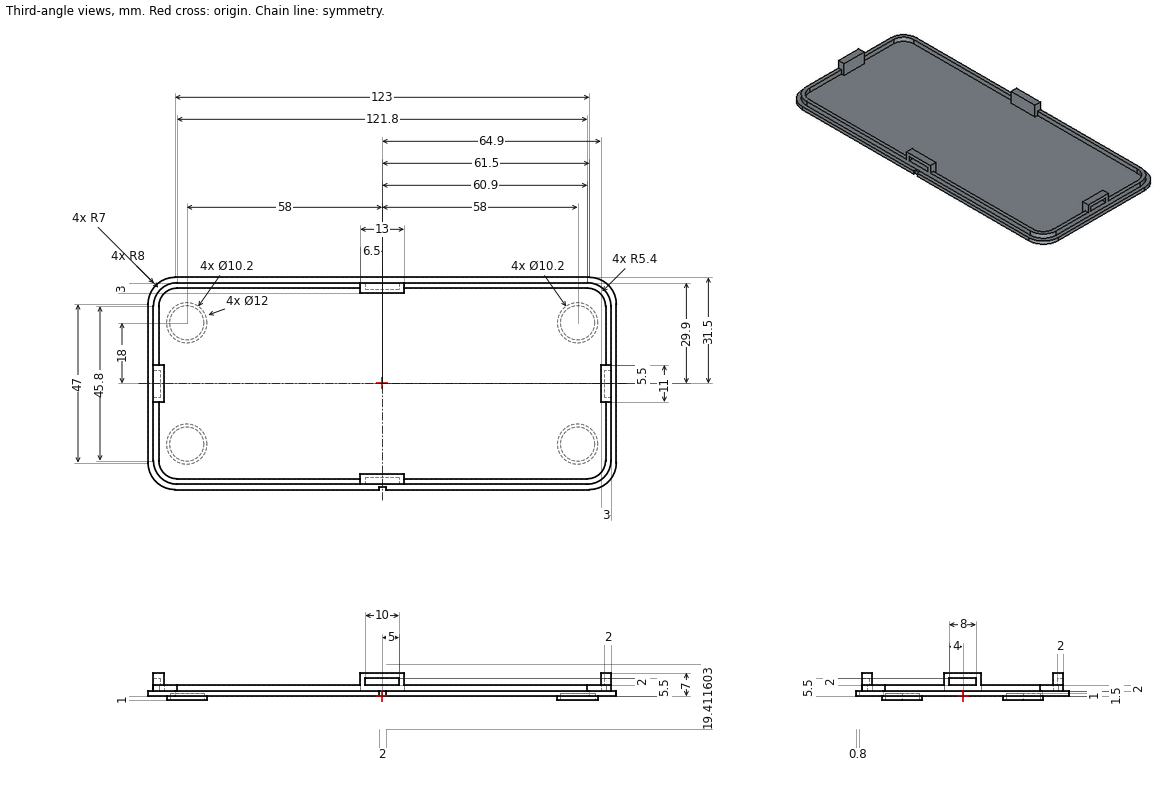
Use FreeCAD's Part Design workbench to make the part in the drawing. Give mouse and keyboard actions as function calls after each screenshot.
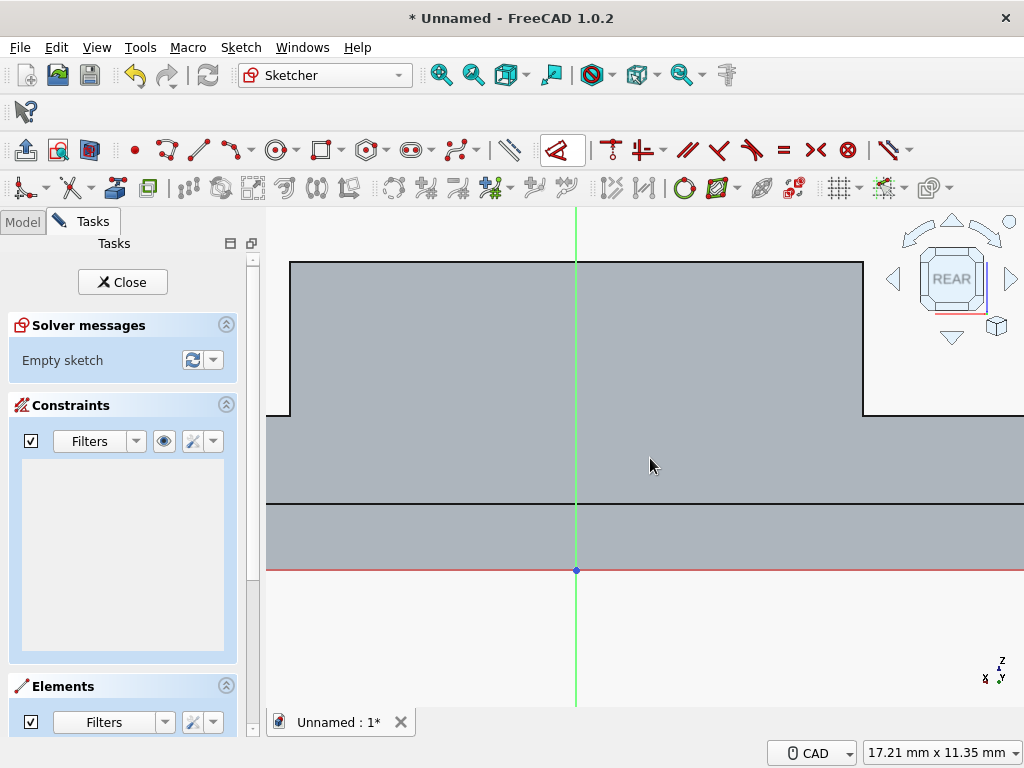
key(g)
key(r)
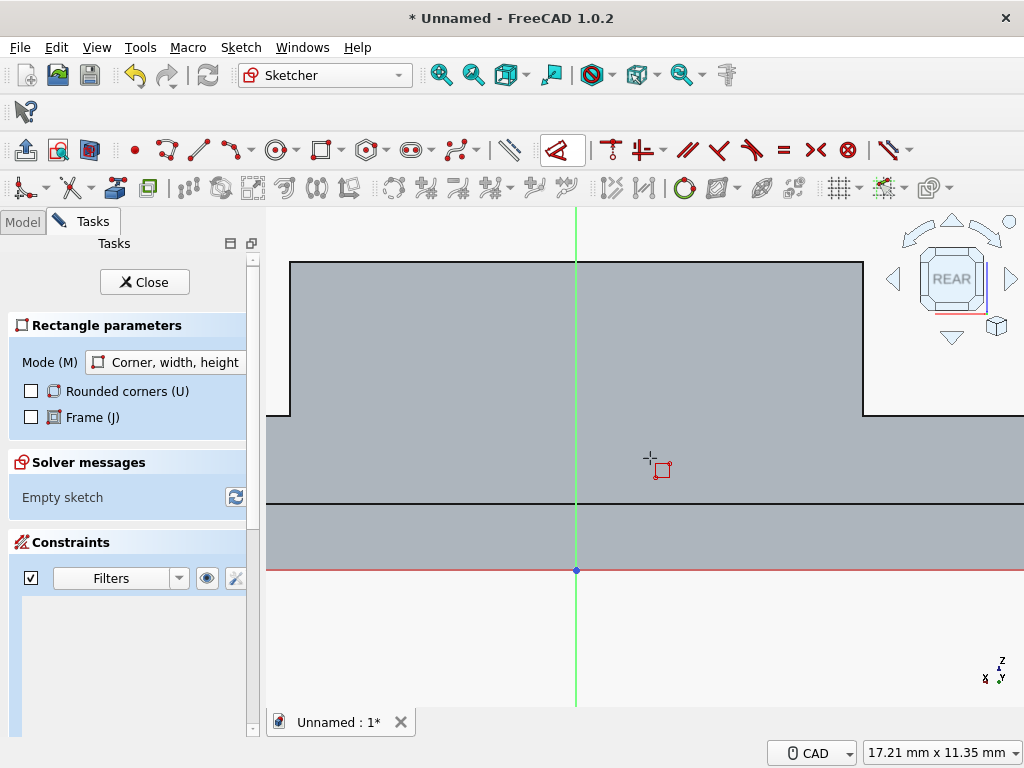
click(356, 328)
click(797, 416)
key(Escape)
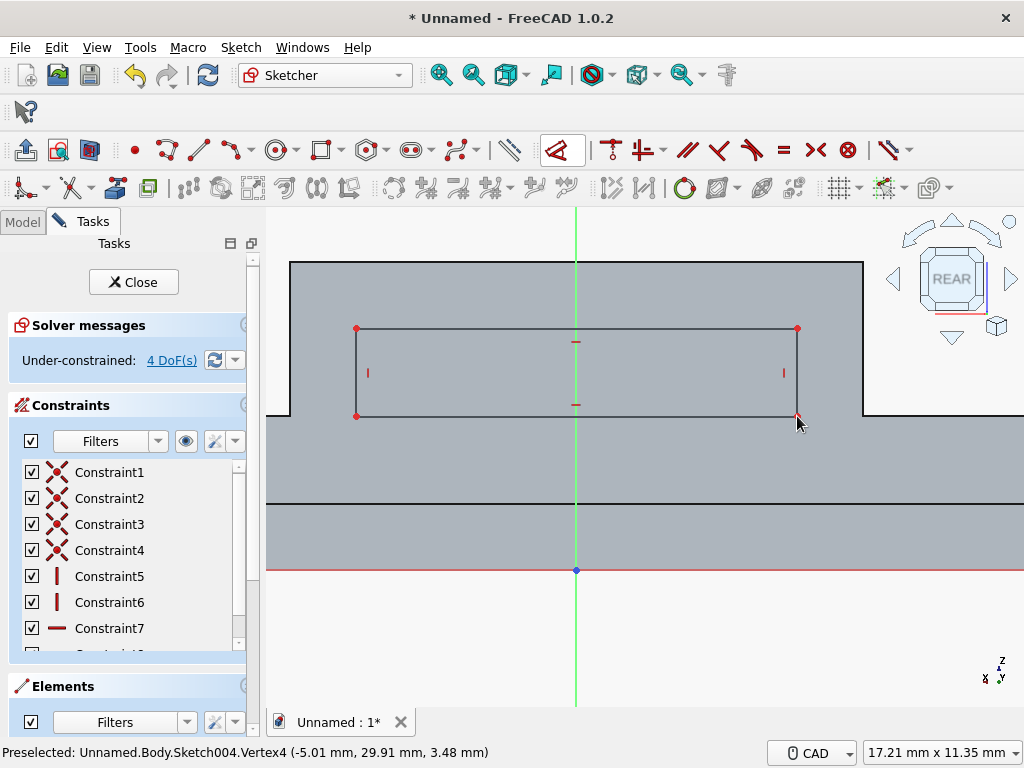
click(356, 355)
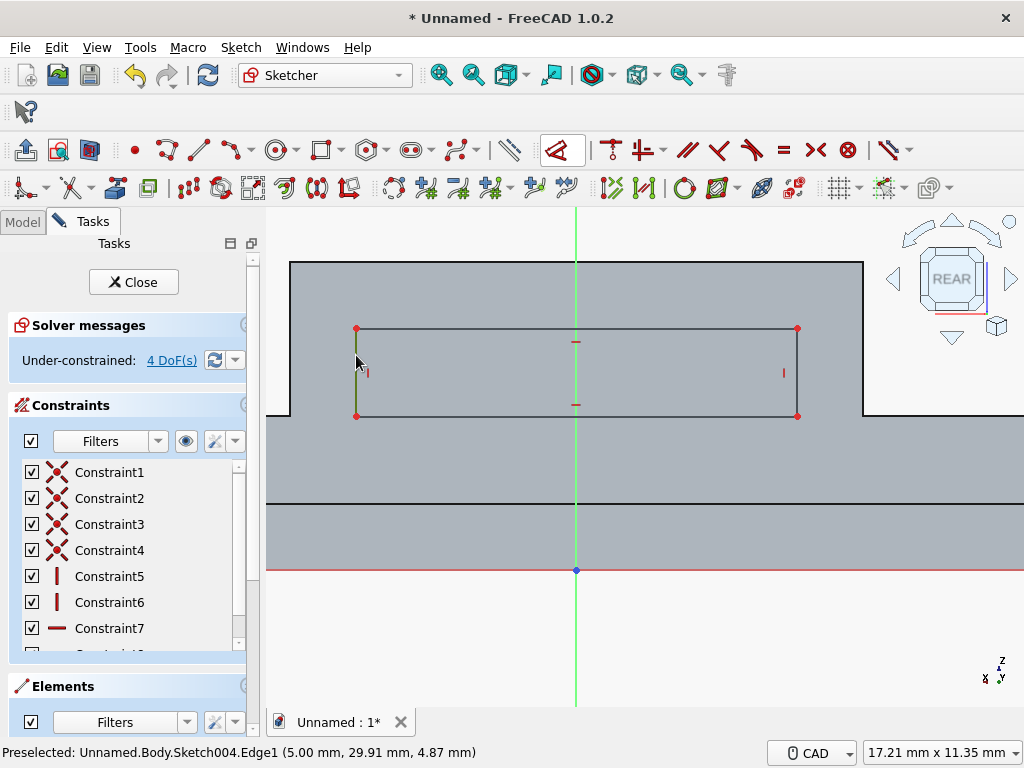
key(i)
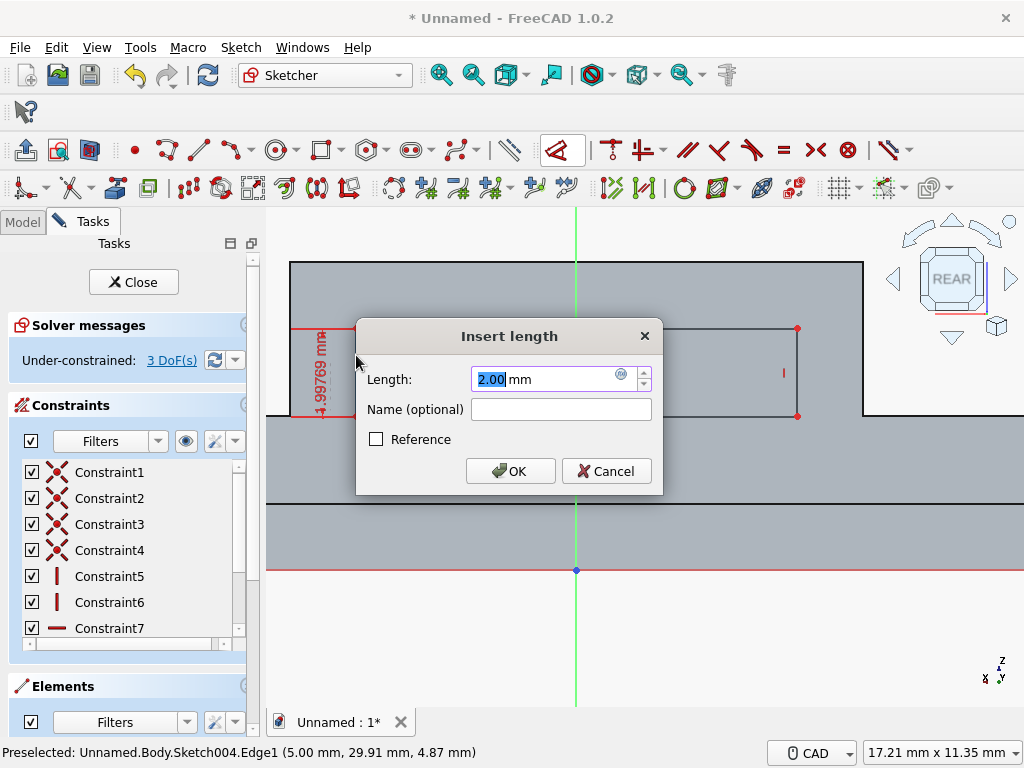
text(2)
key(Return)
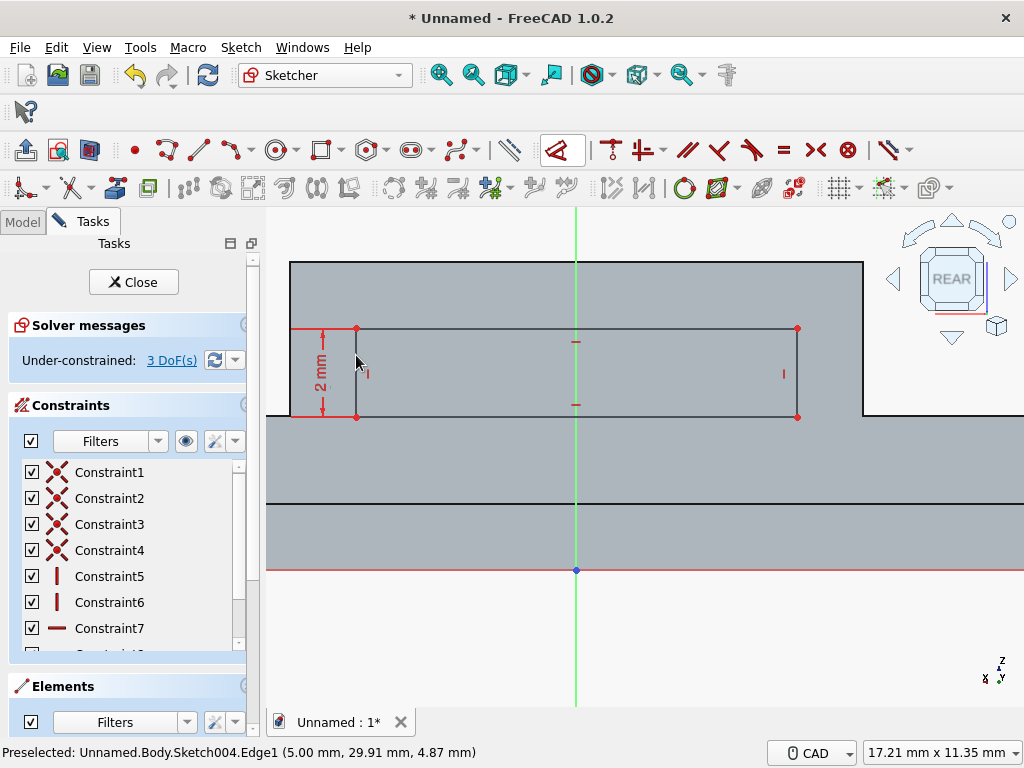
click(488, 417)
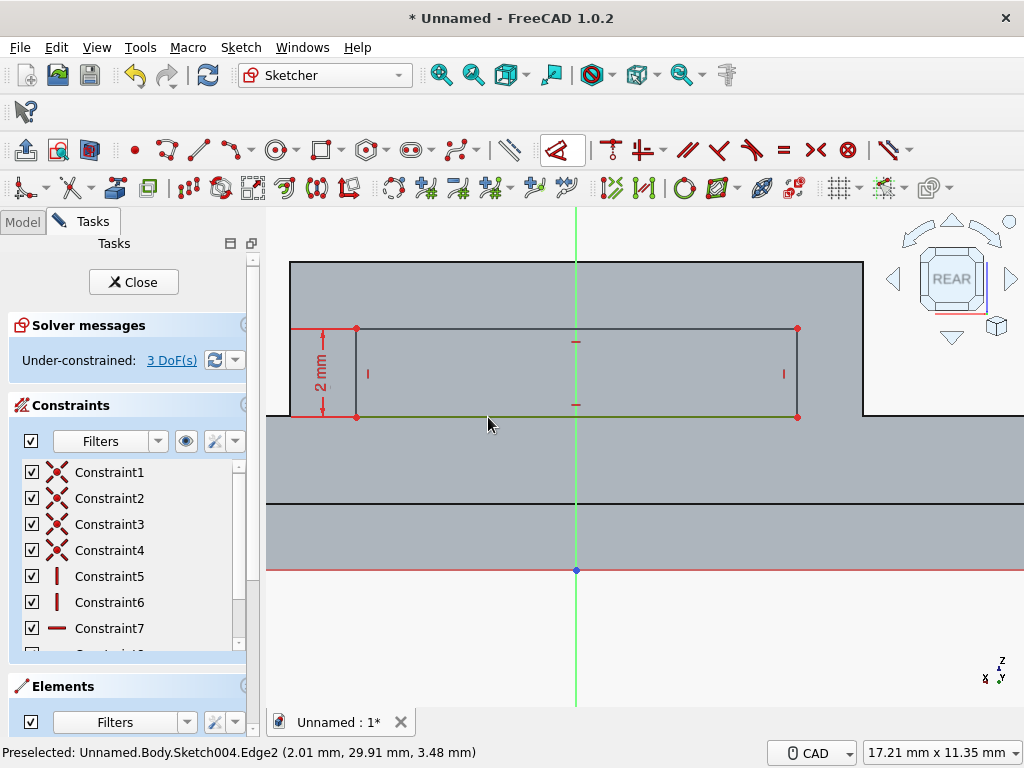
key(l)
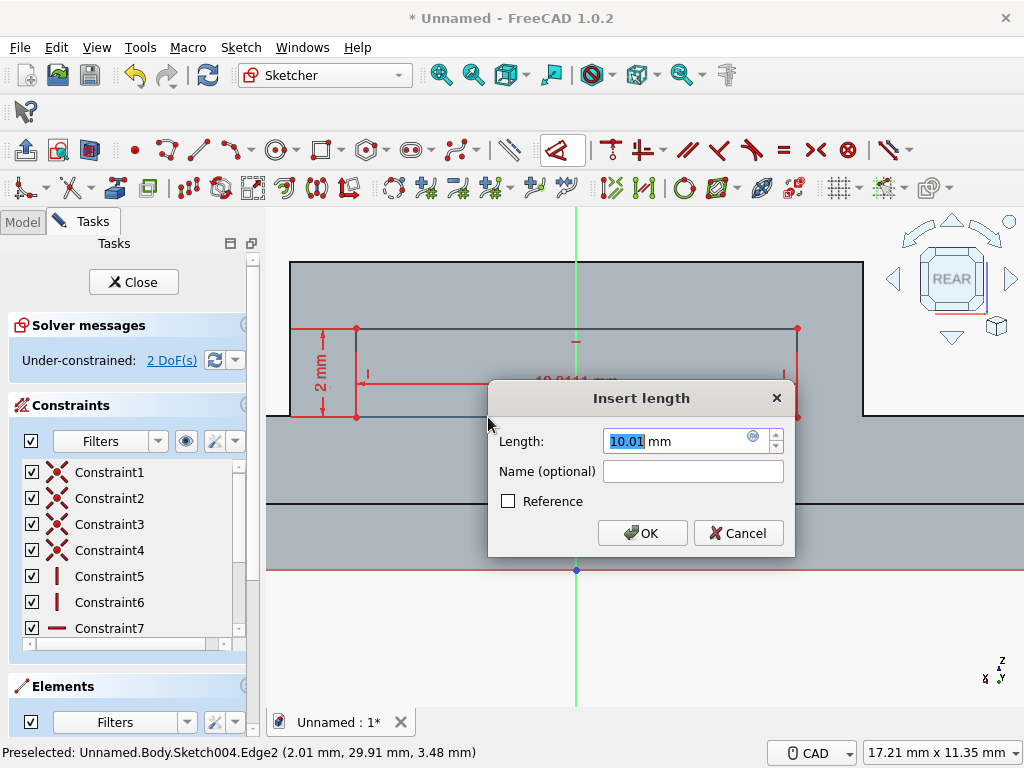
text(10)
key(Return)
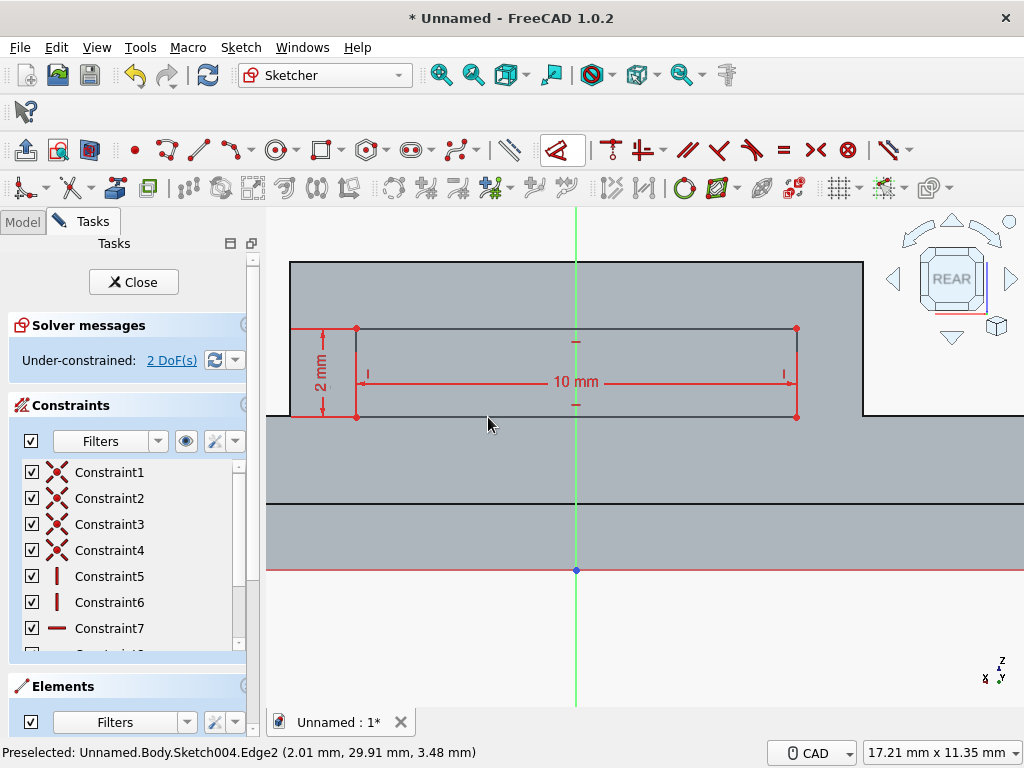
click(356, 329)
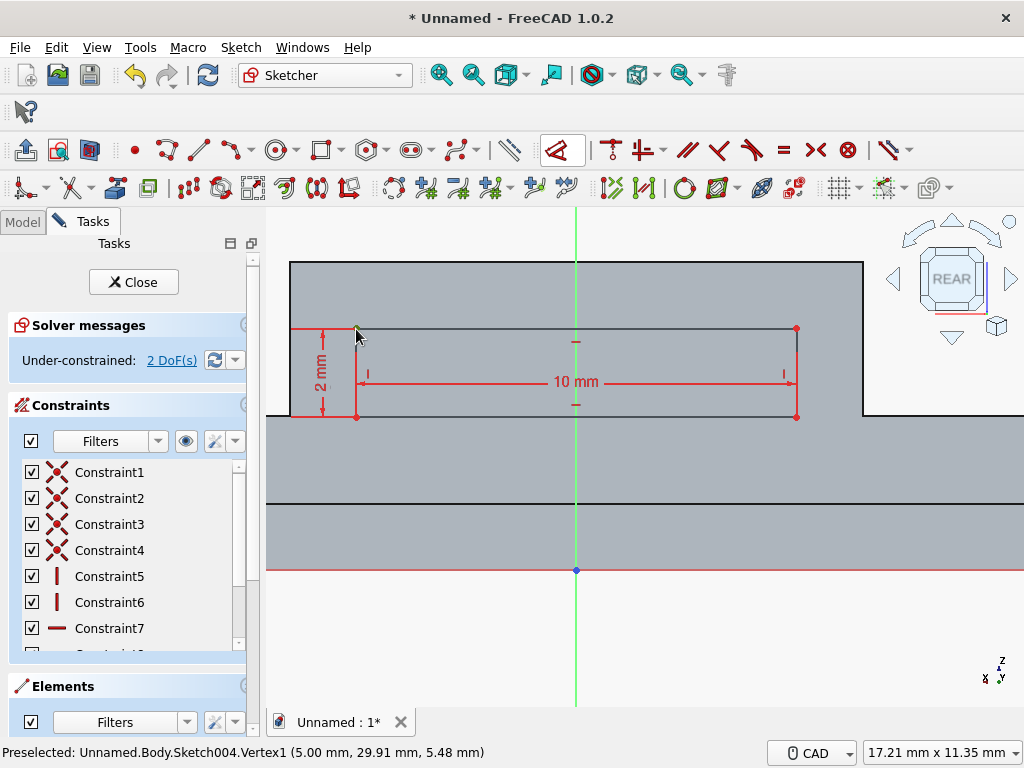
key(l)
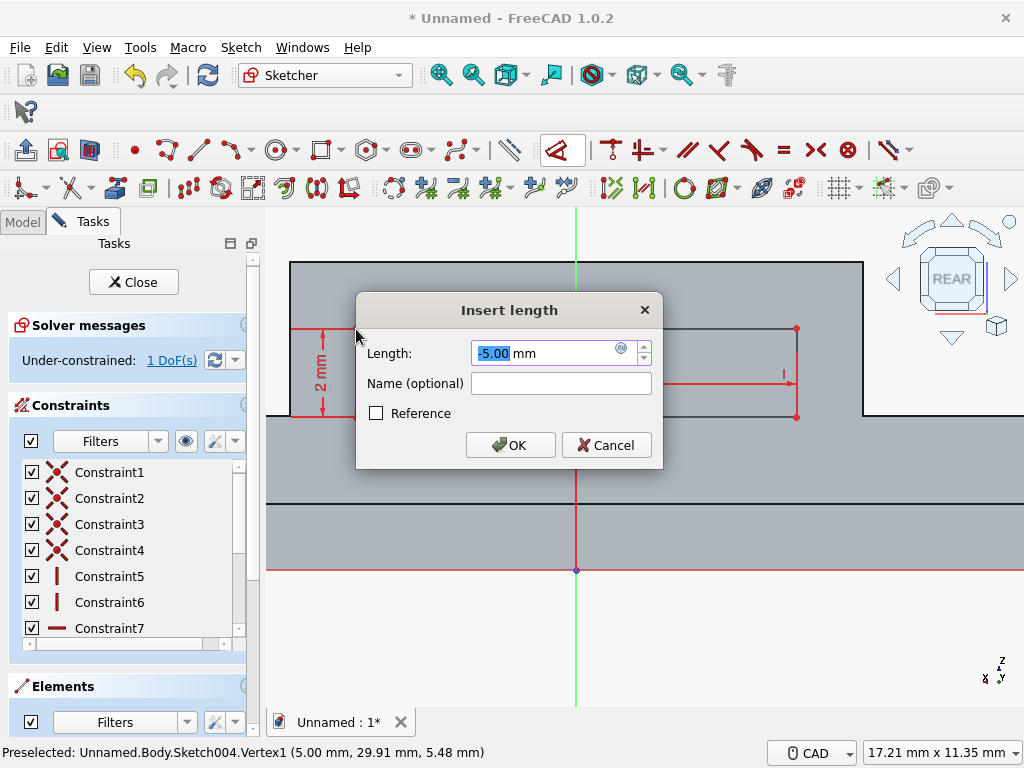
text(-5)
key(Return)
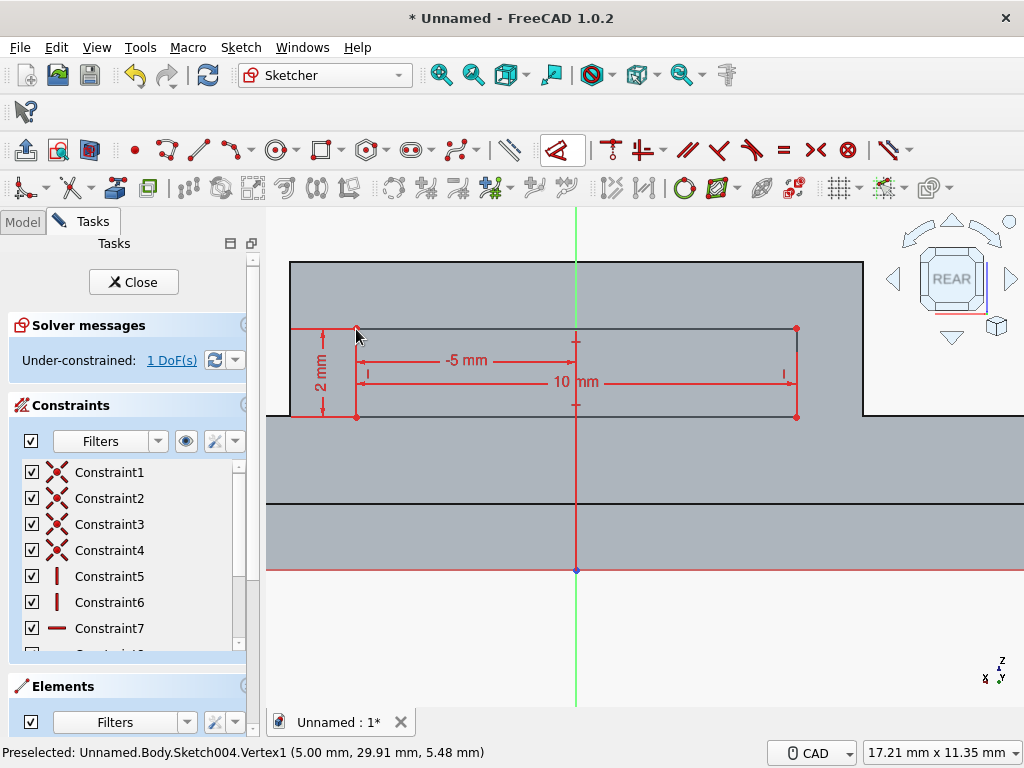
click(356, 329)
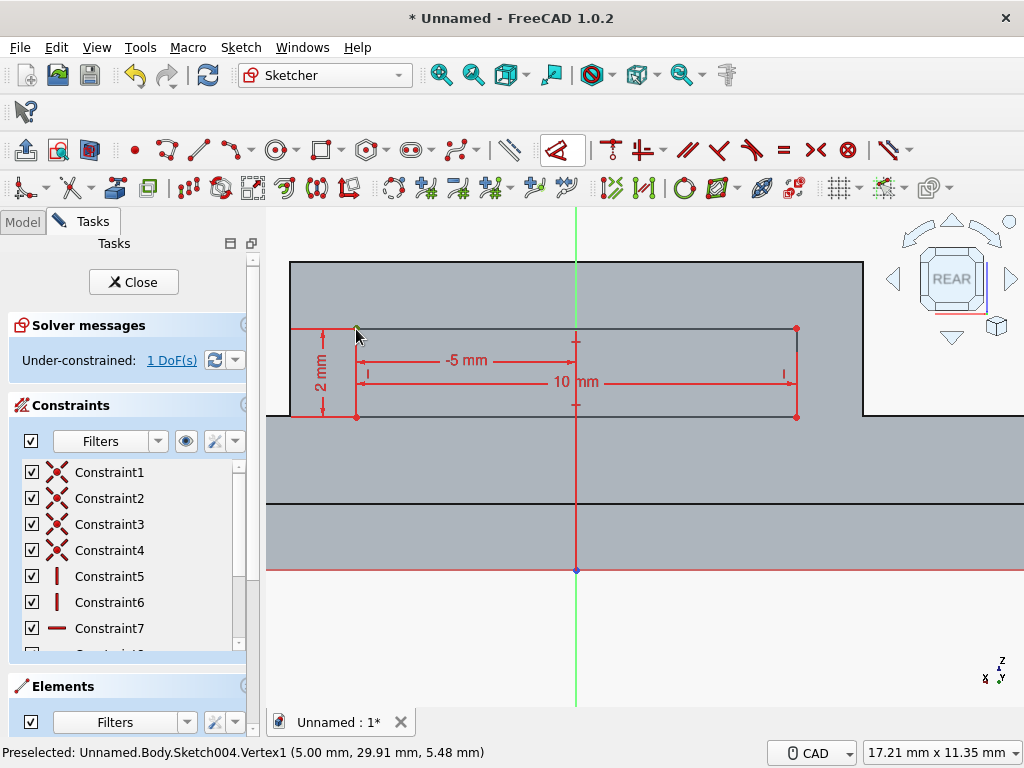
key(i)